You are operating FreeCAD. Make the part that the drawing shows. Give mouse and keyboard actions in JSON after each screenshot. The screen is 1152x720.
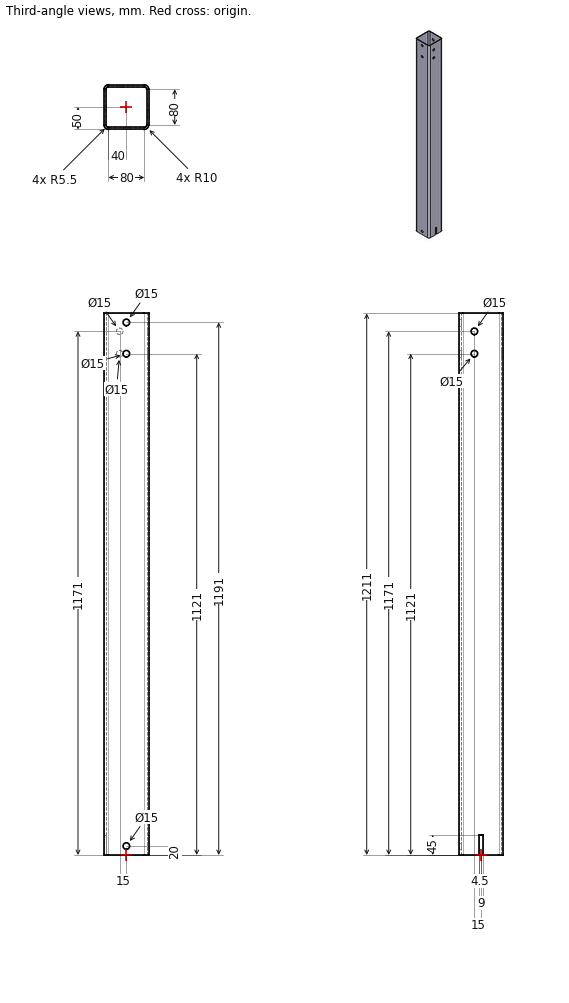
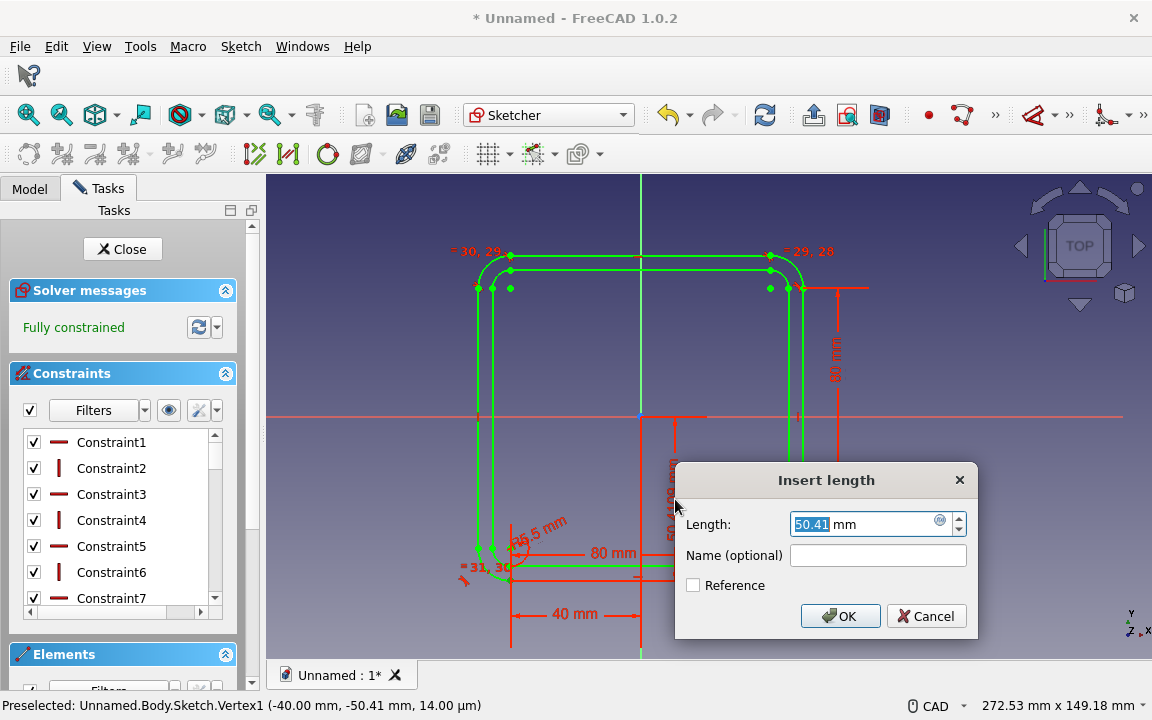
{"action": "type", "text": "50"}
{"action": "key", "text": "Return"}
{"action": "key", "text": "Escape"}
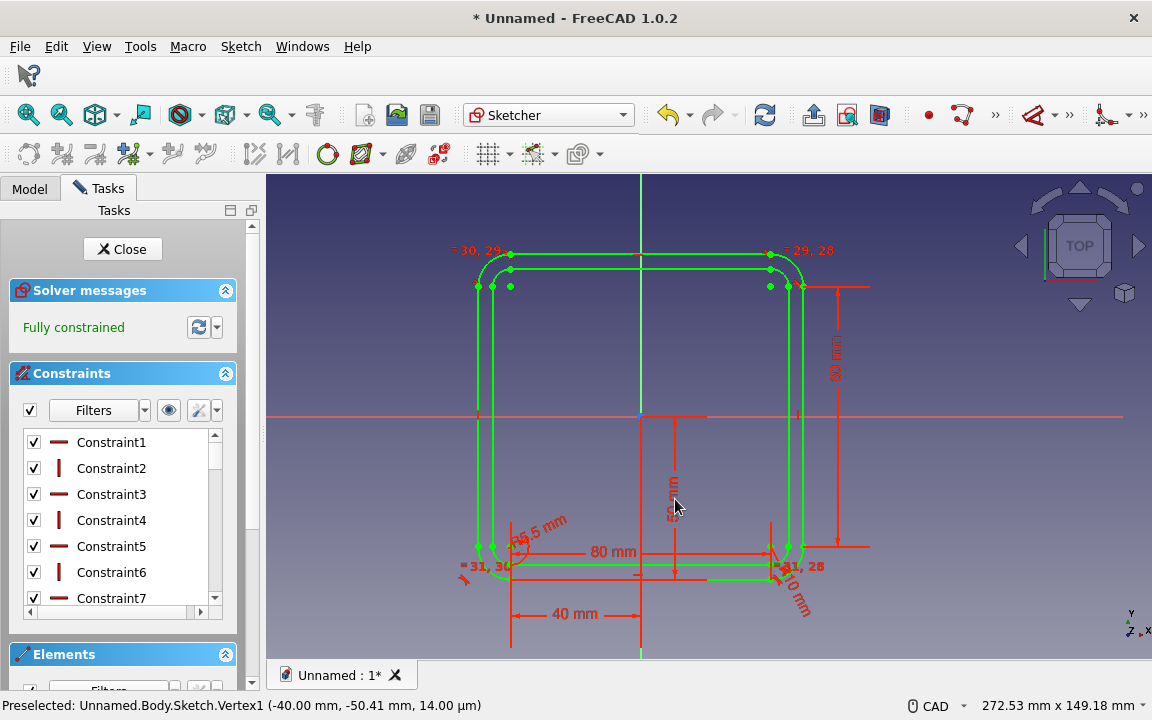
{"action": "left_click", "coordinate": [123, 249]}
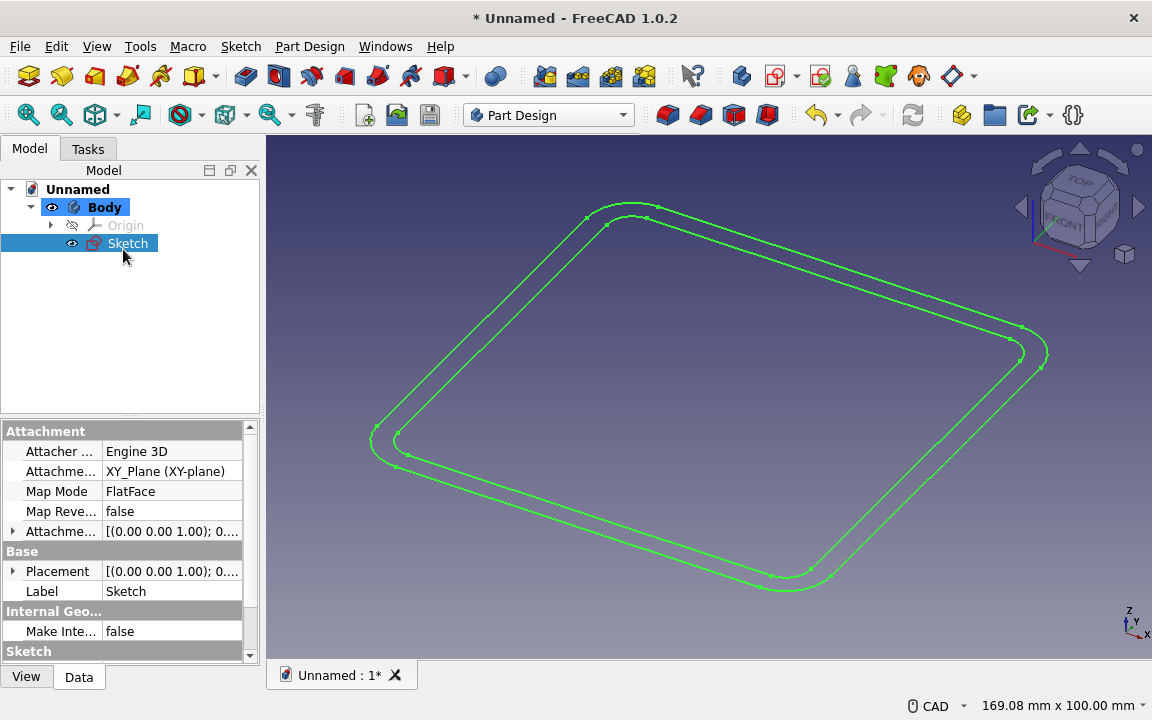
{"action": "left_click", "coordinate": [29, 76]}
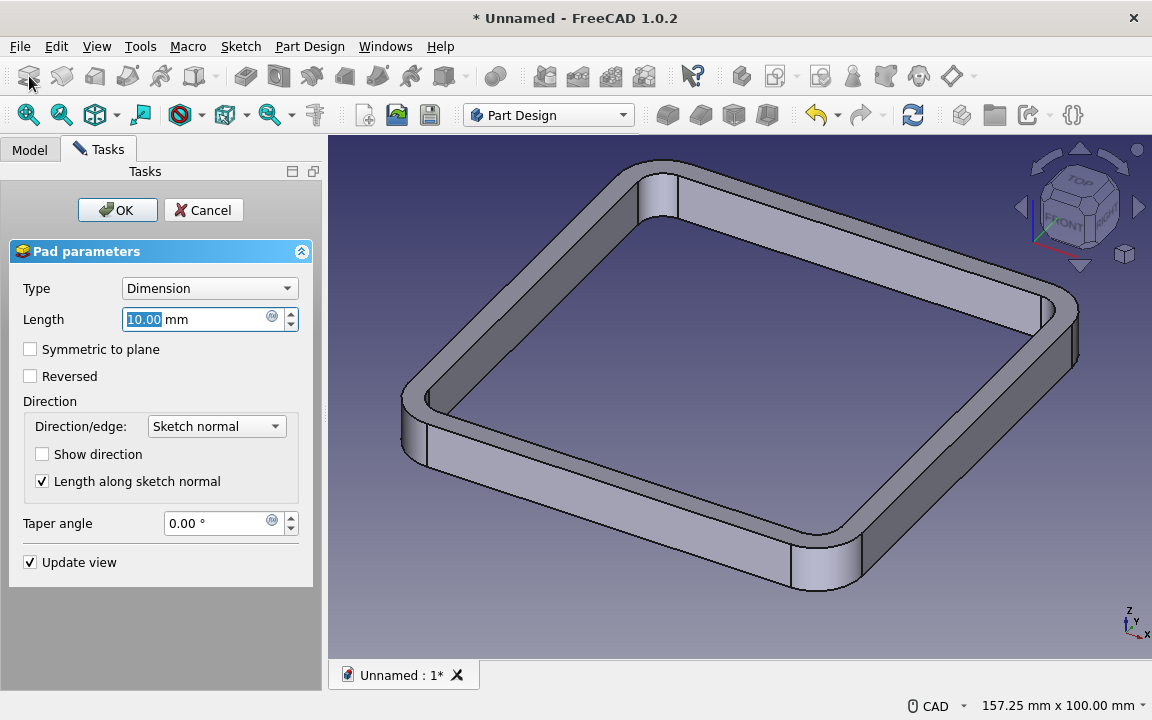
{"action": "type", "text": "1211"}
{"action": "key", "text": "Tab"}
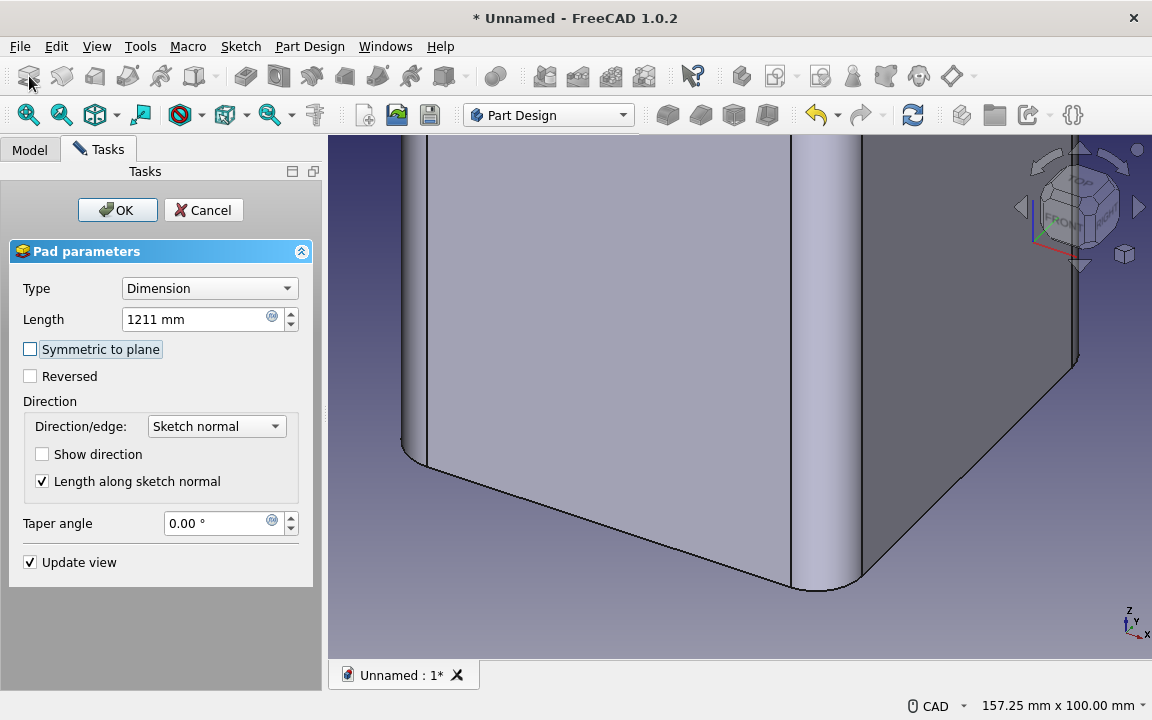
{"action": "left_click", "coordinate": [118, 210]}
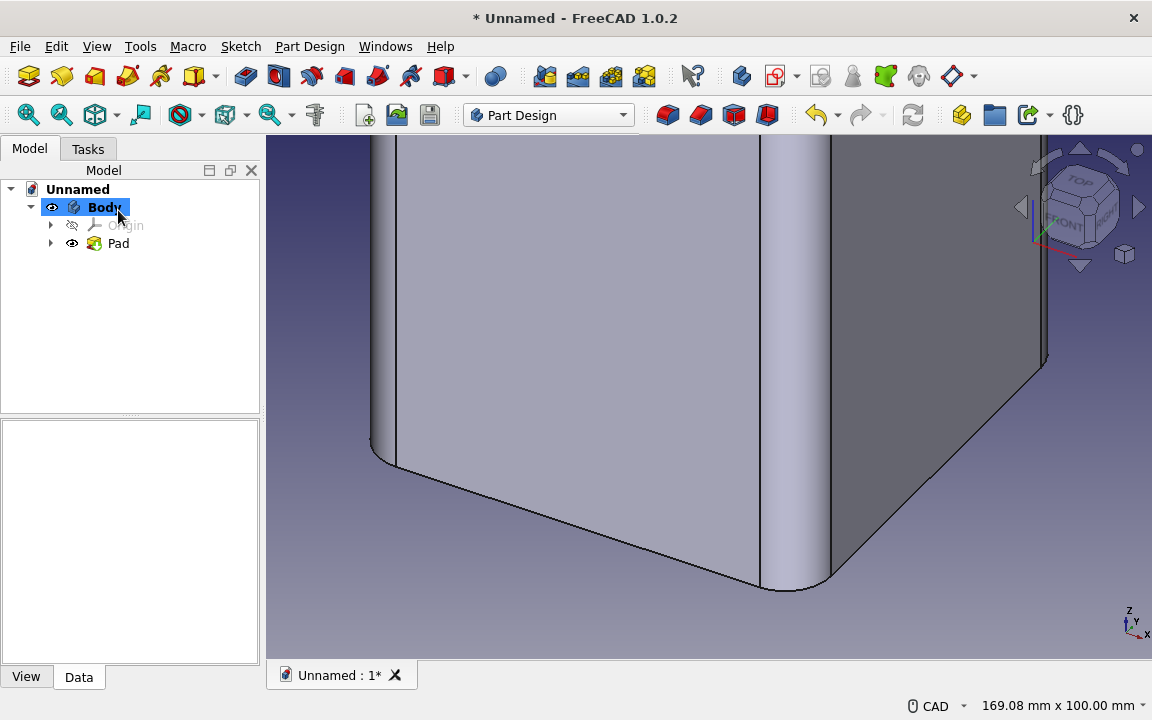
{"action": "left_click", "coordinate": [29, 116]}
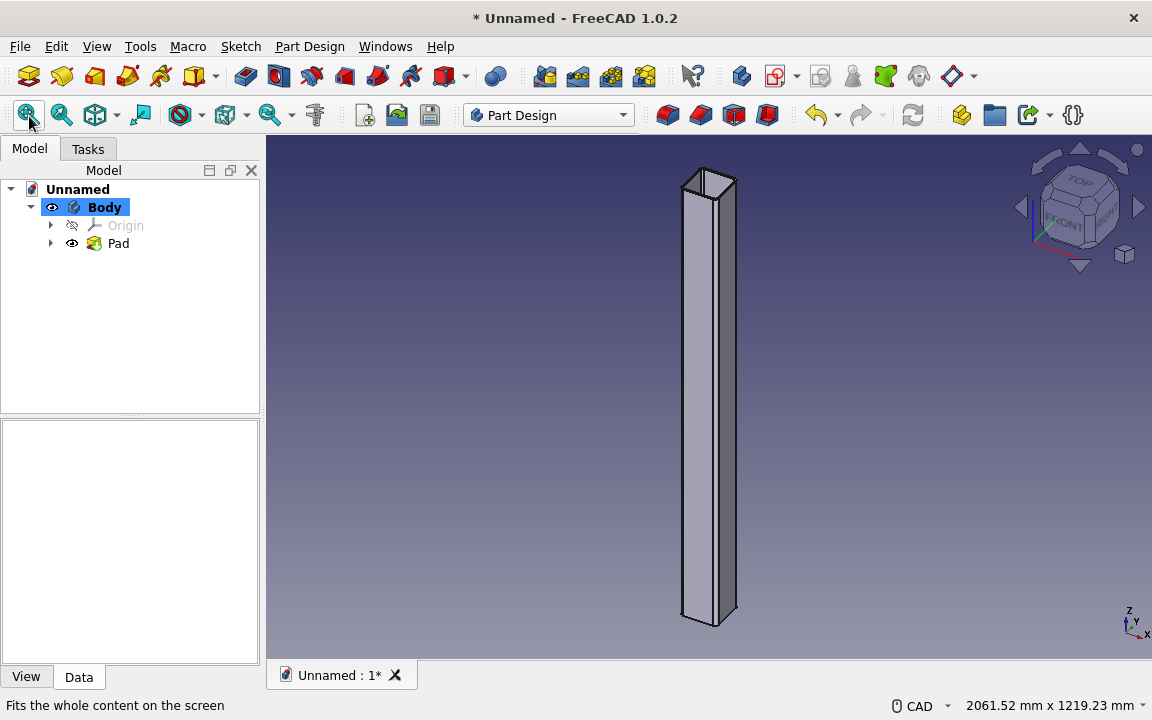
{"action": "left_click", "coordinate": [728, 219]}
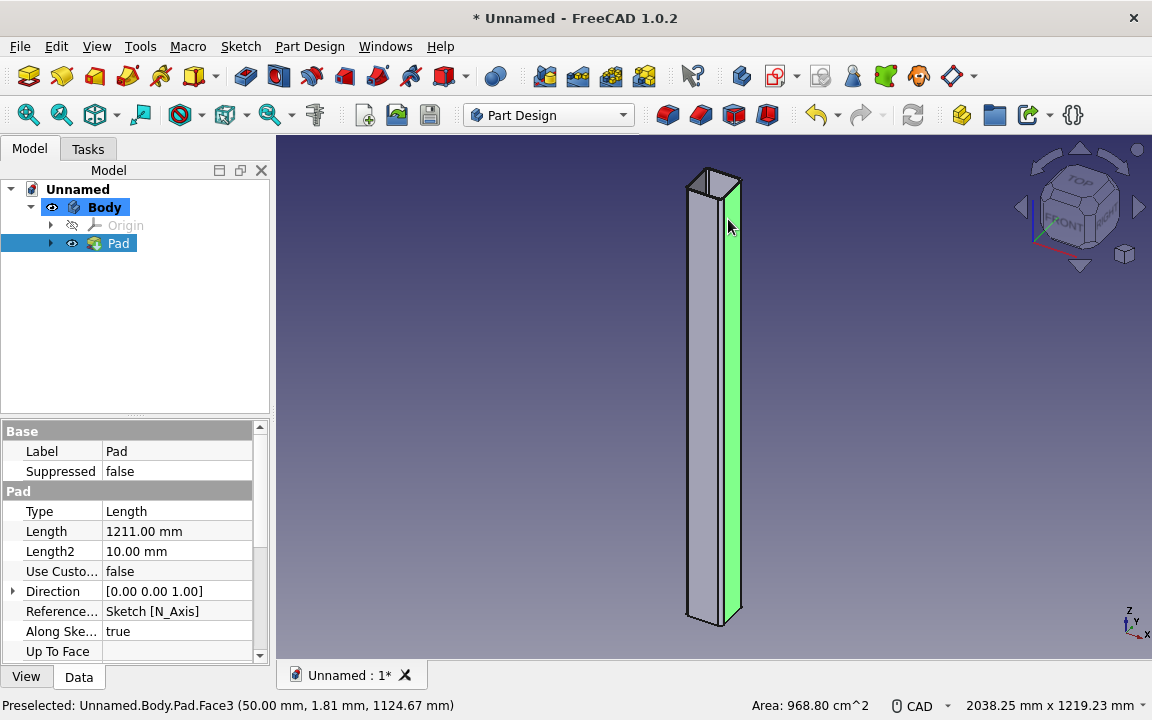
{"action": "left_click", "coordinate": [774, 76]}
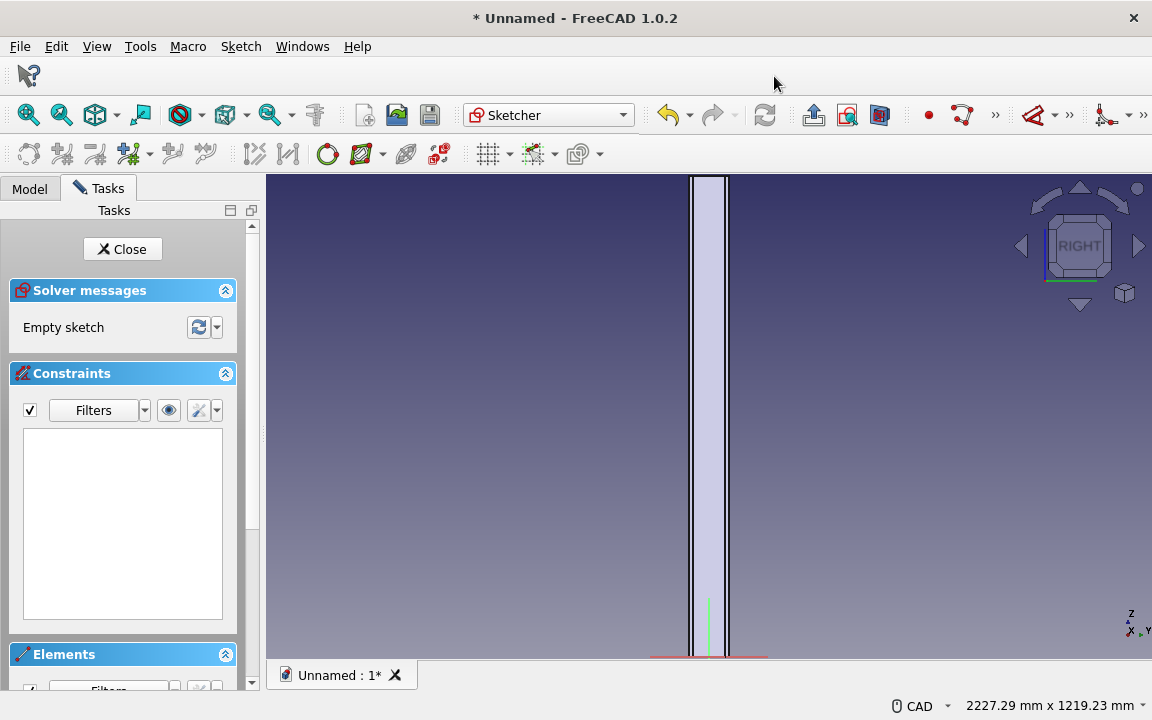
{"action": "scroll", "coordinate": [640, 416], "scroll_direction": "down", "scroll_amount": 5}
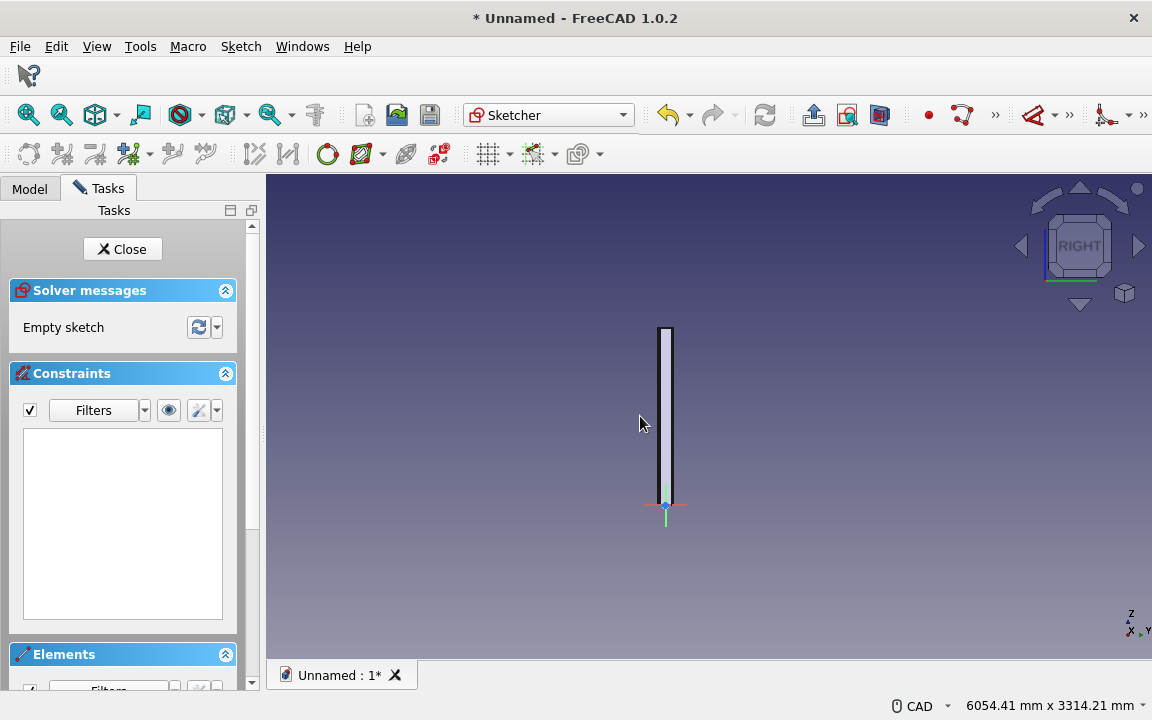
{"action": "scroll", "coordinate": [665, 329], "scroll_direction": "up", "scroll_amount": 15}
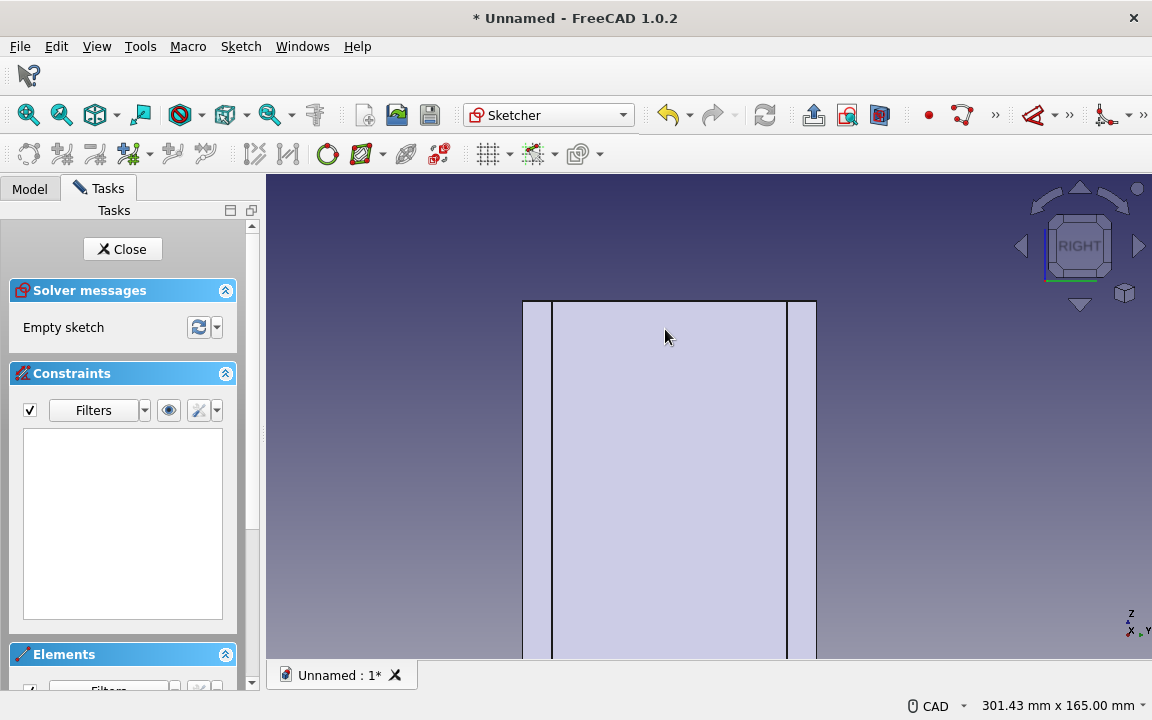
{"action": "scroll", "coordinate": [623, 418], "scroll_direction": "up", "scroll_amount": 10}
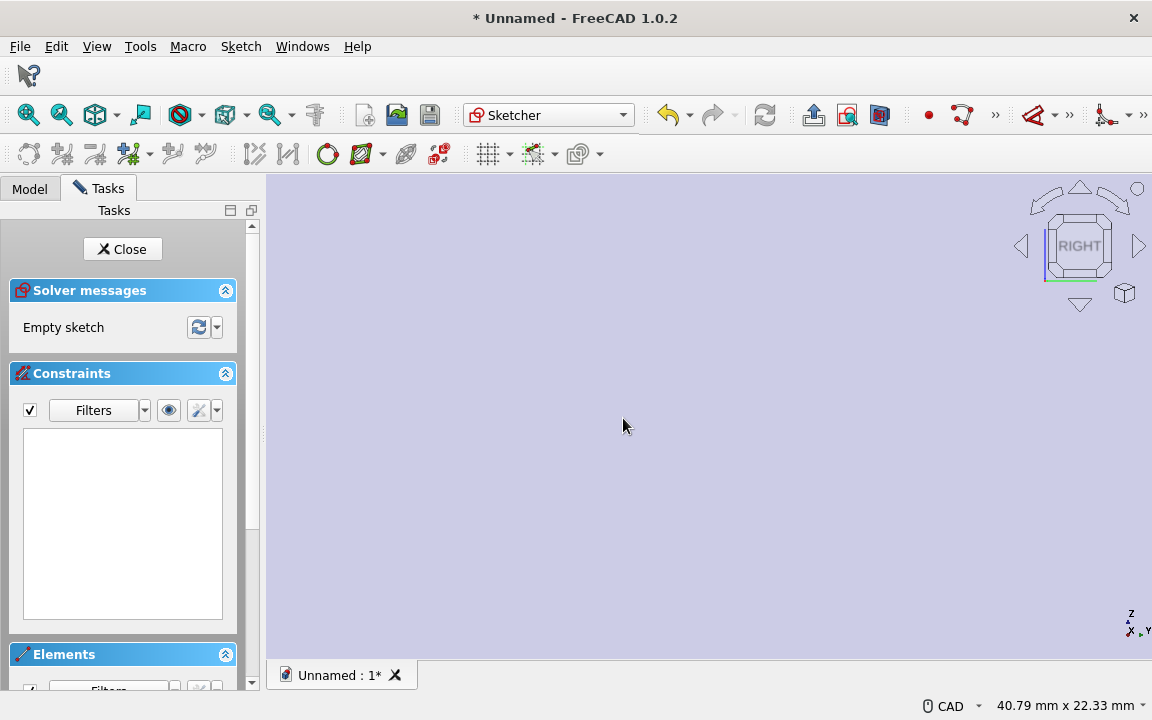
{"action": "key", "text": "g c"}